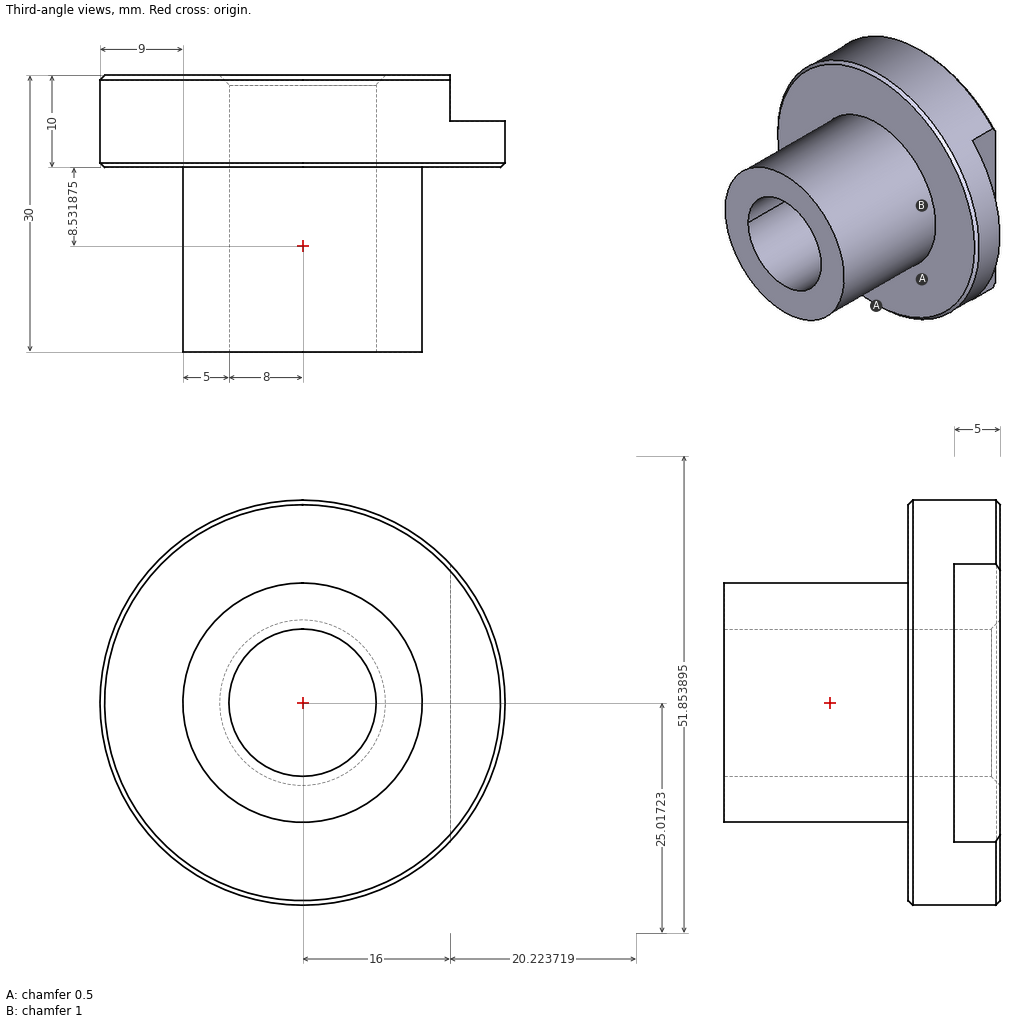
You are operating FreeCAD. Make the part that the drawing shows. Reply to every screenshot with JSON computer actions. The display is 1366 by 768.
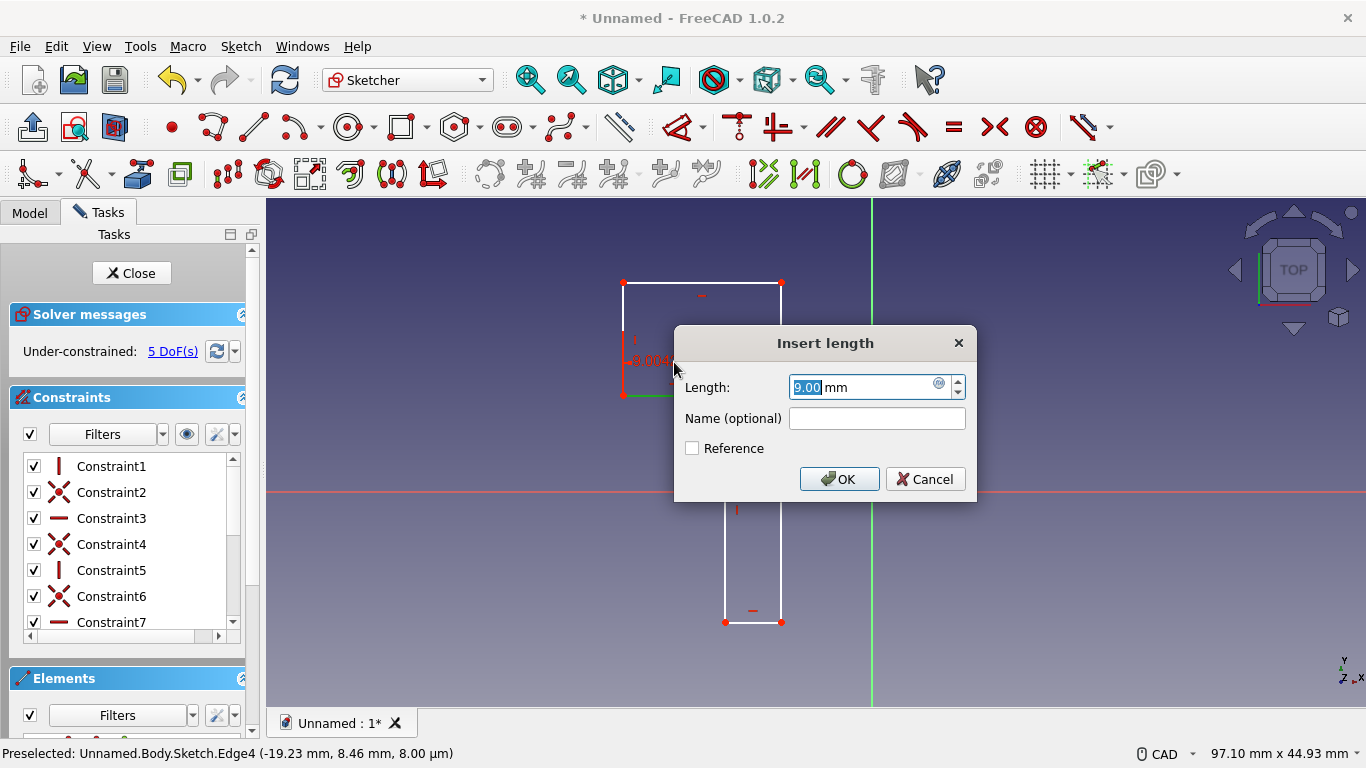
{"action": "type", "text": "9"}
{"action": "key", "text": "Return"}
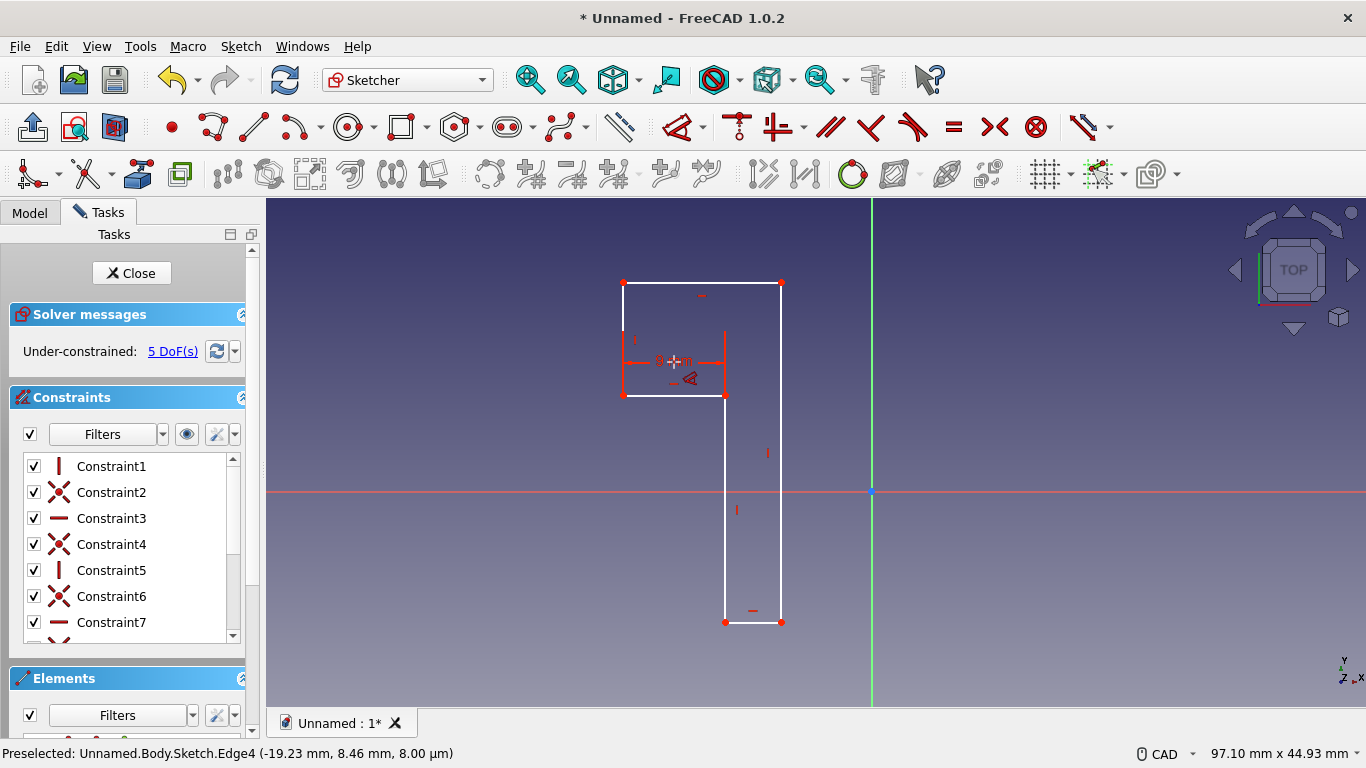
{"action": "left_click", "coordinate": [742, 623]}
{"action": "left_click", "coordinate": [753, 657]}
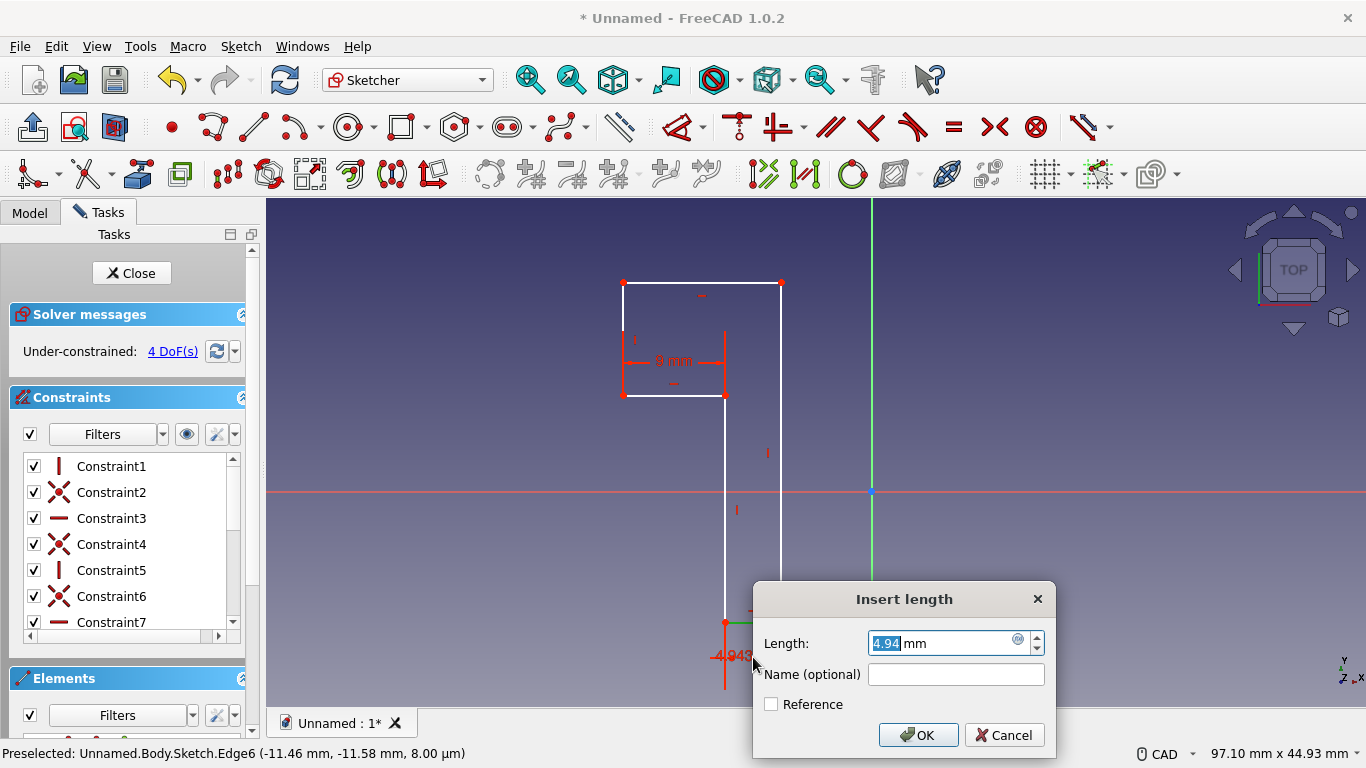
{"action": "type", "text": "5"}
{"action": "key", "text": "Return"}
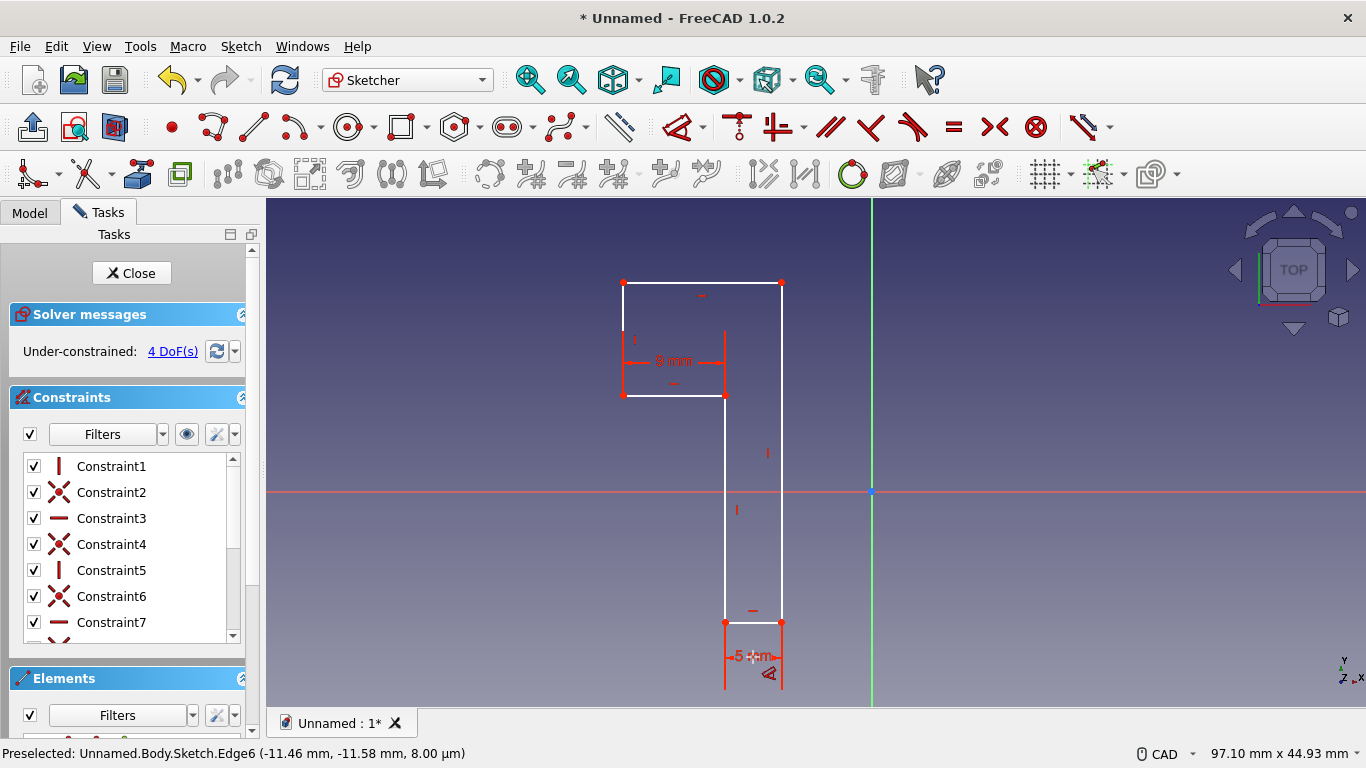
{"action": "left_click", "coordinate": [782, 521]}
{"action": "left_click", "coordinate": [816, 453]}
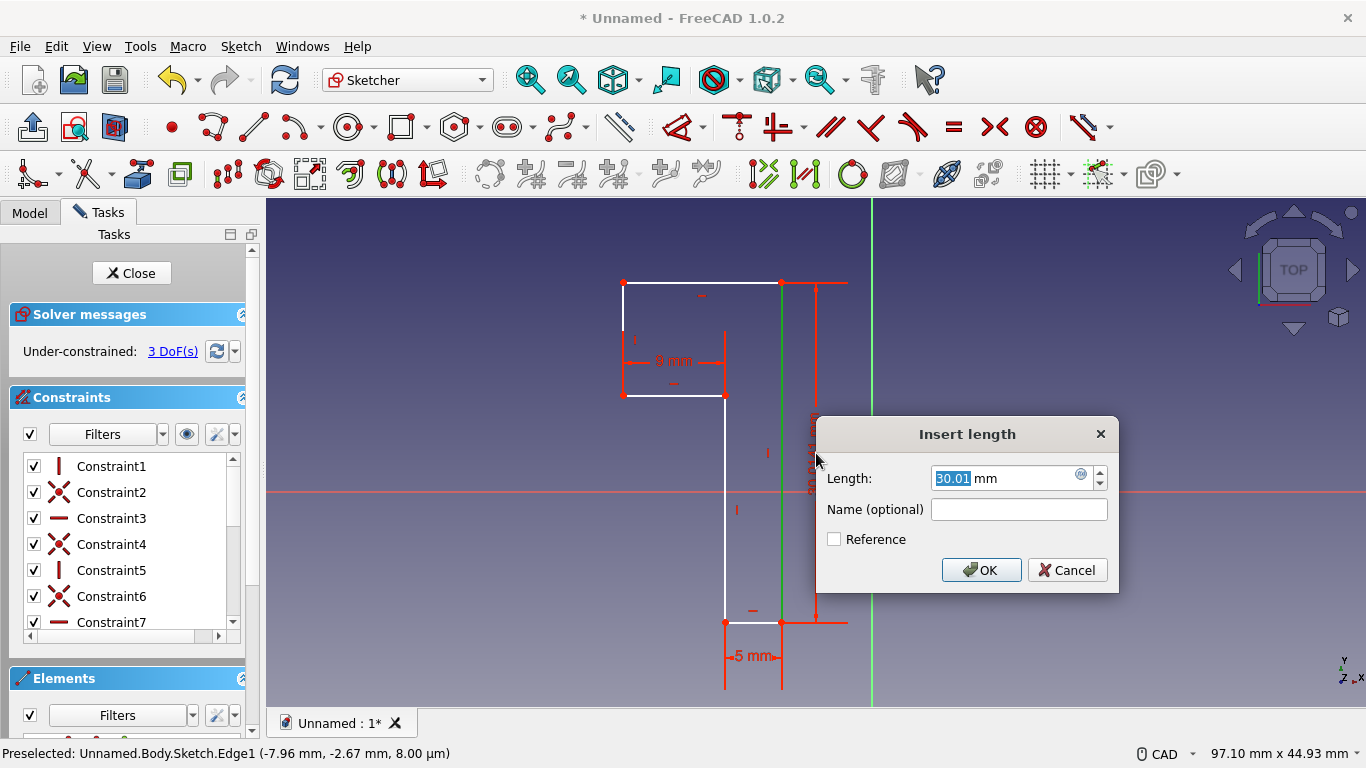
{"action": "type", "text": "30"}
{"action": "key", "text": "Return"}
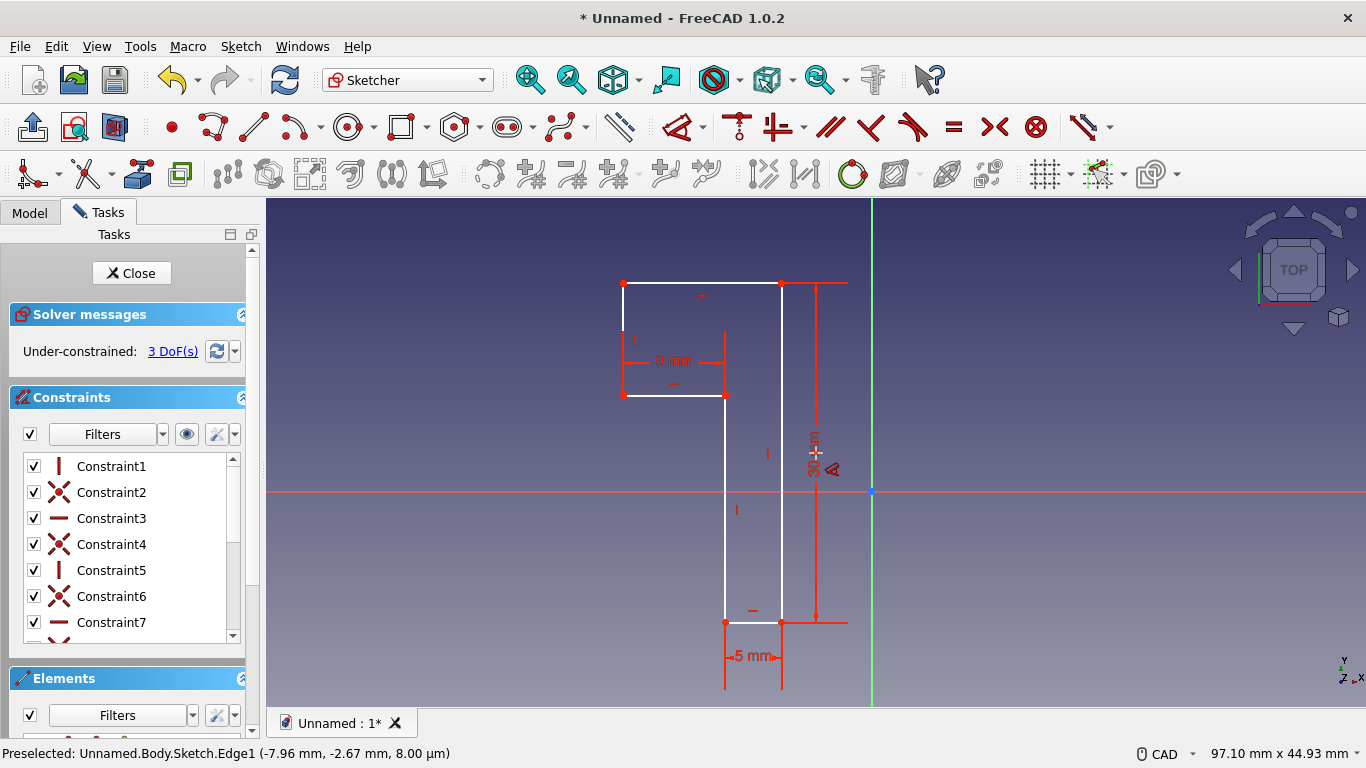
{"action": "left_click", "coordinate": [623, 317]}
{"action": "left_click", "coordinate": [589, 340]}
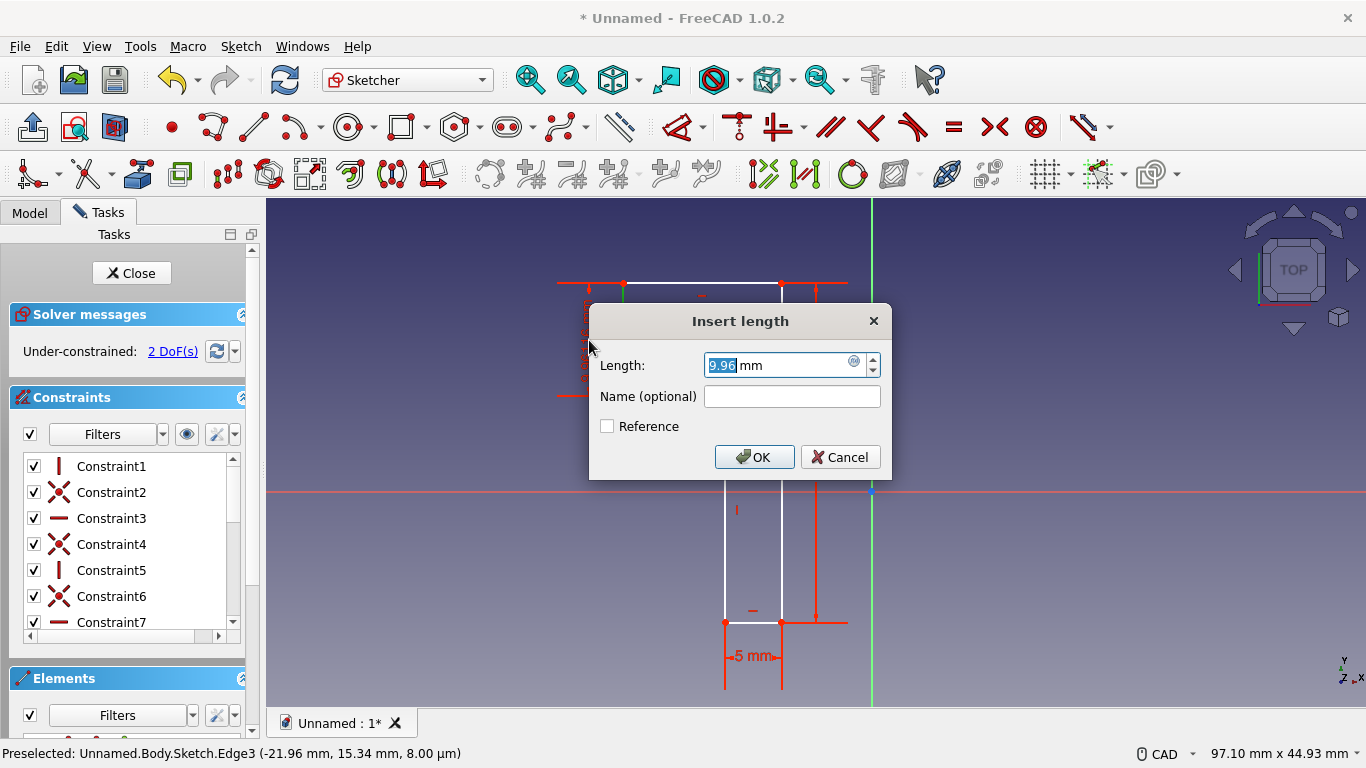
{"action": "type", "text": "10"}
{"action": "key", "text": "Return"}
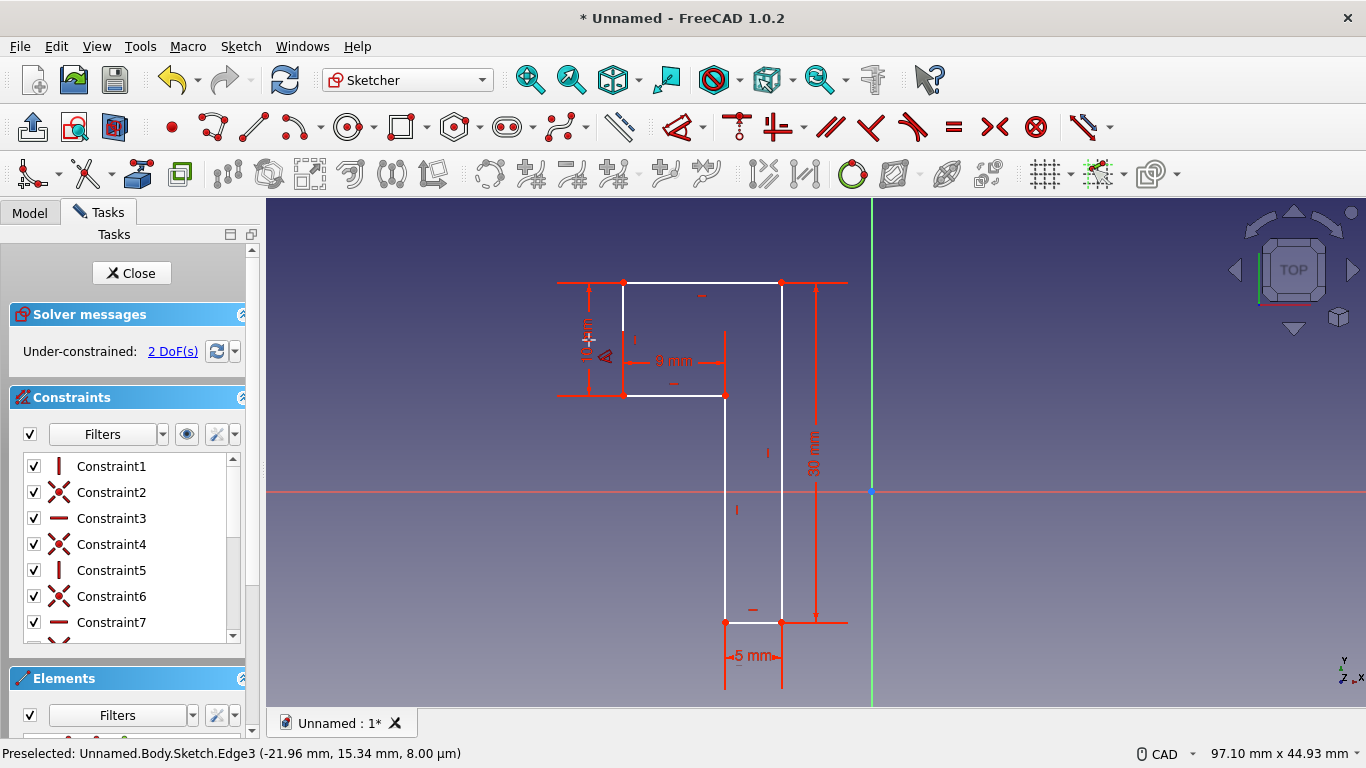
{"action": "left_click", "coordinate": [782, 623]}
{"action": "left_click", "coordinate": [827, 657]}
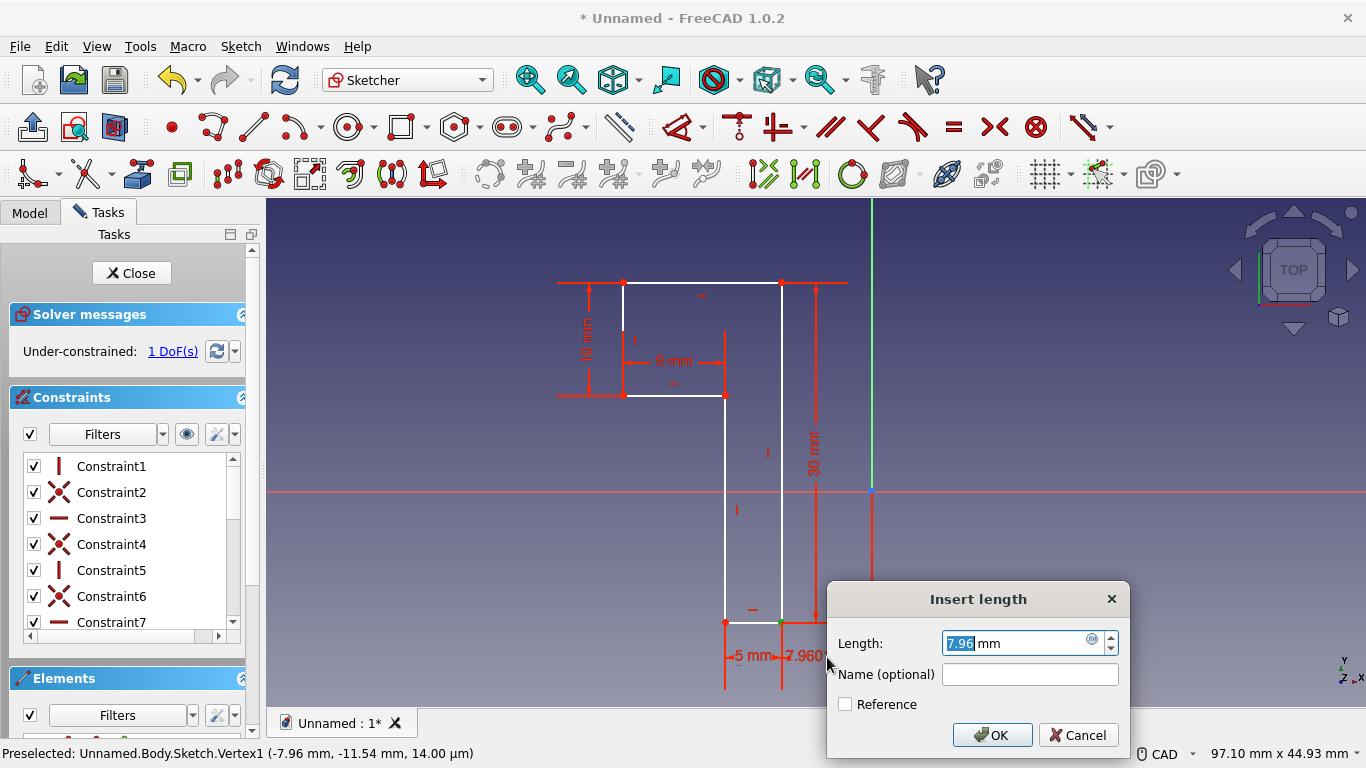
{"action": "type", "text": "8"}
{"action": "key", "text": "Return"}